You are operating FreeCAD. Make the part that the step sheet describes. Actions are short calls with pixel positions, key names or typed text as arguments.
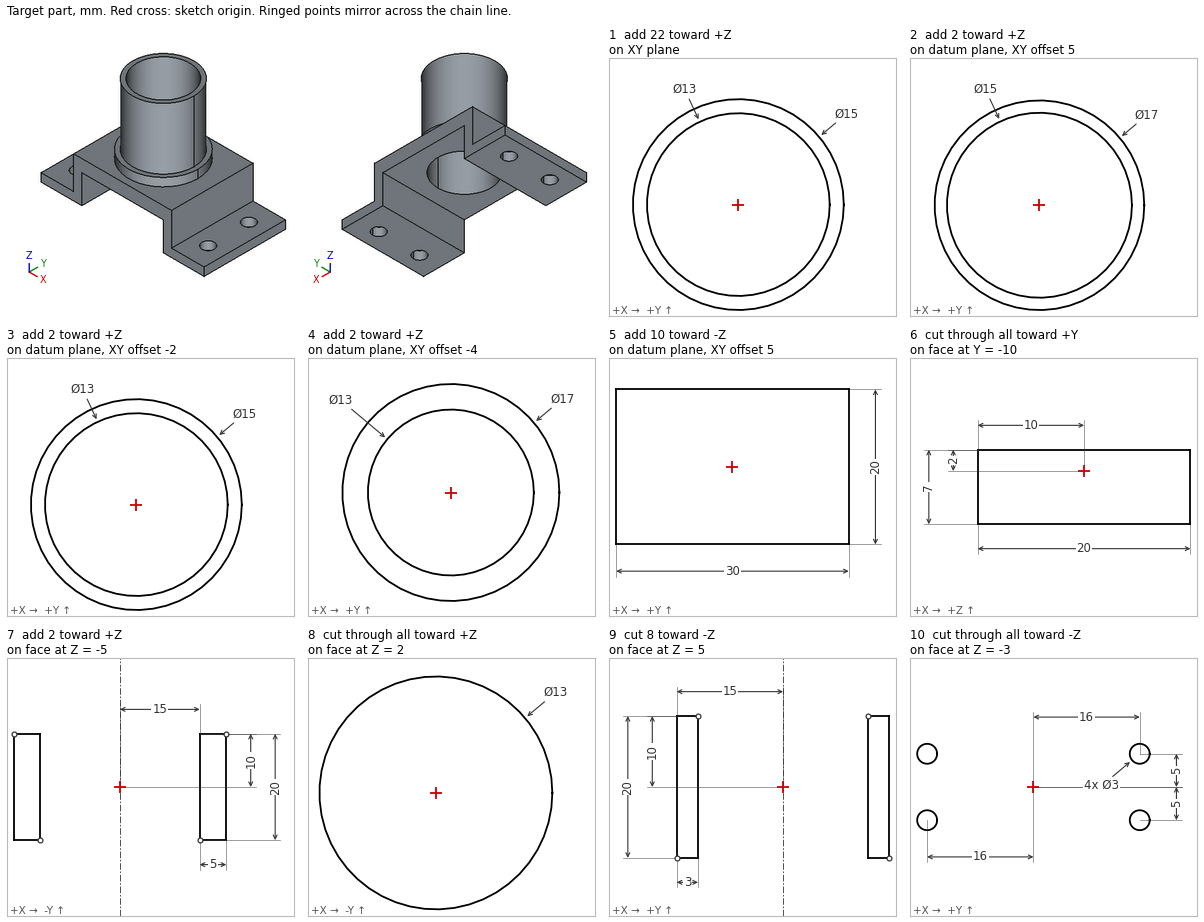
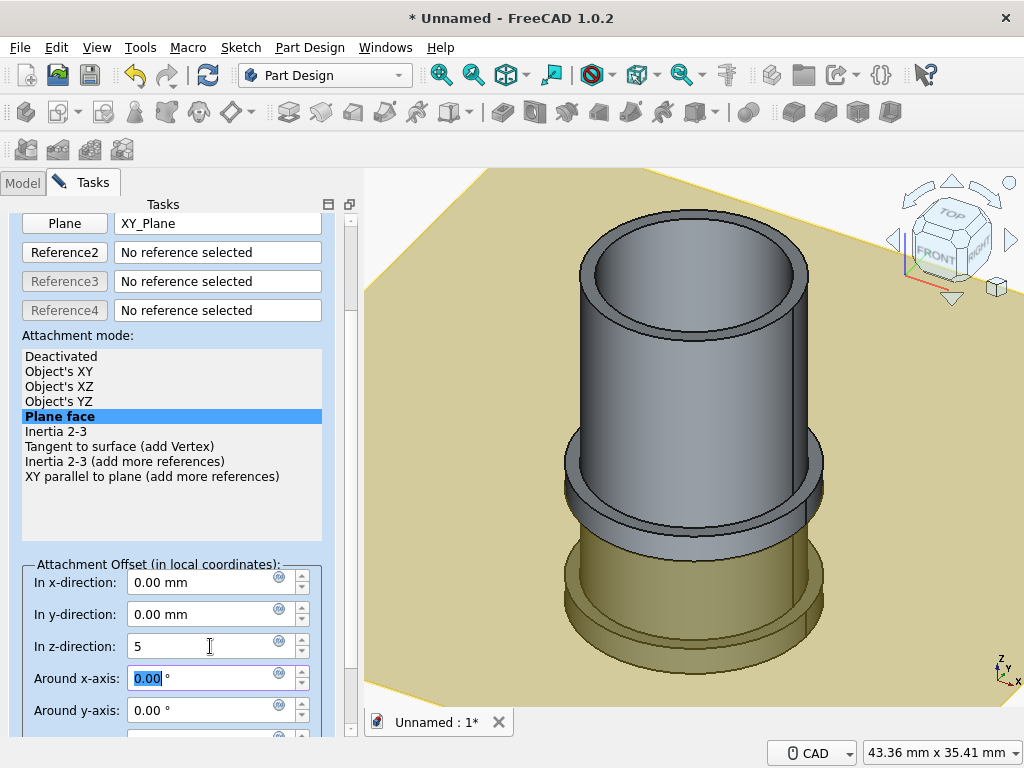
scroll(351, 475, up, 3)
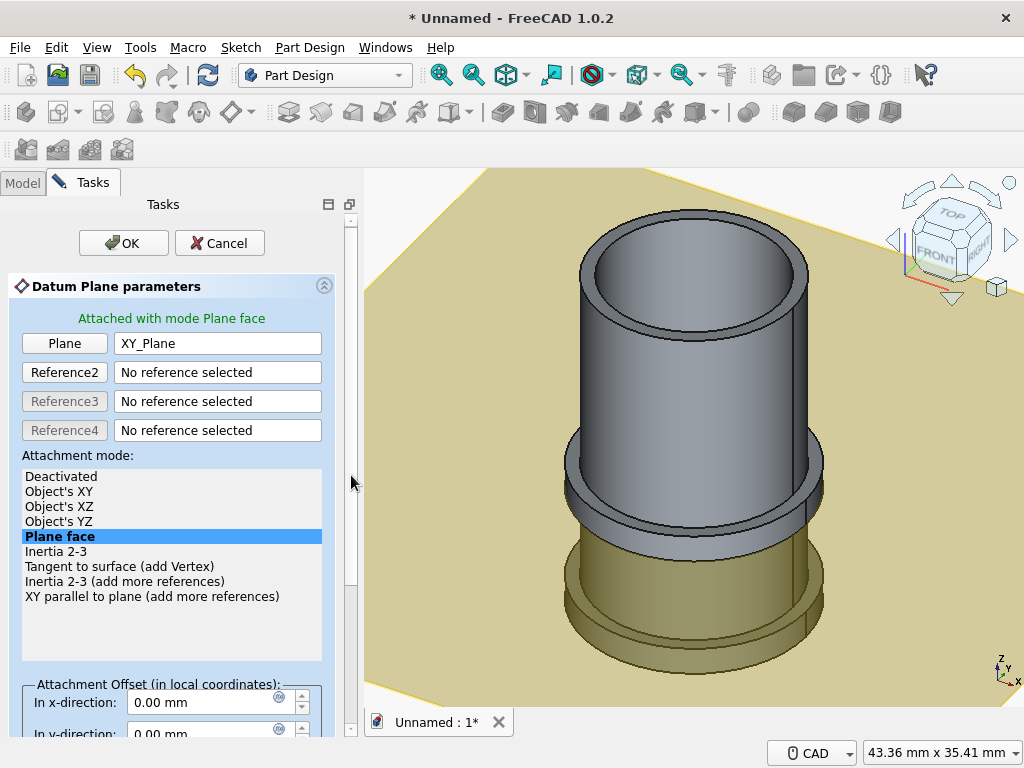
click(124, 243)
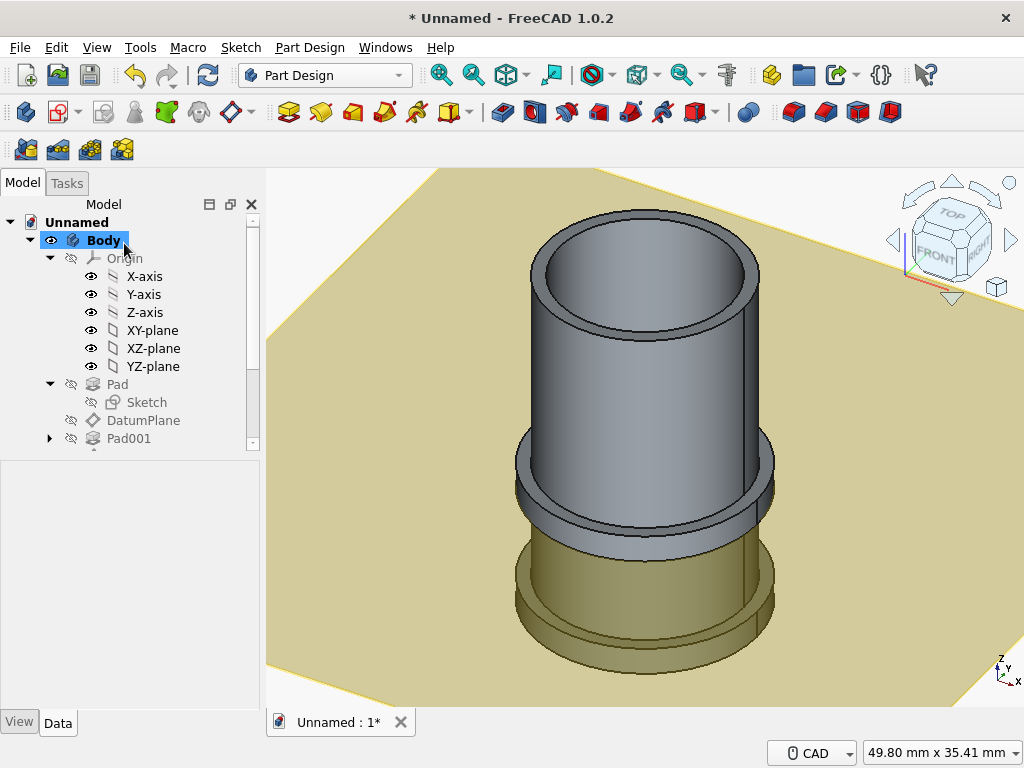
scroll(100, 326, down, 3)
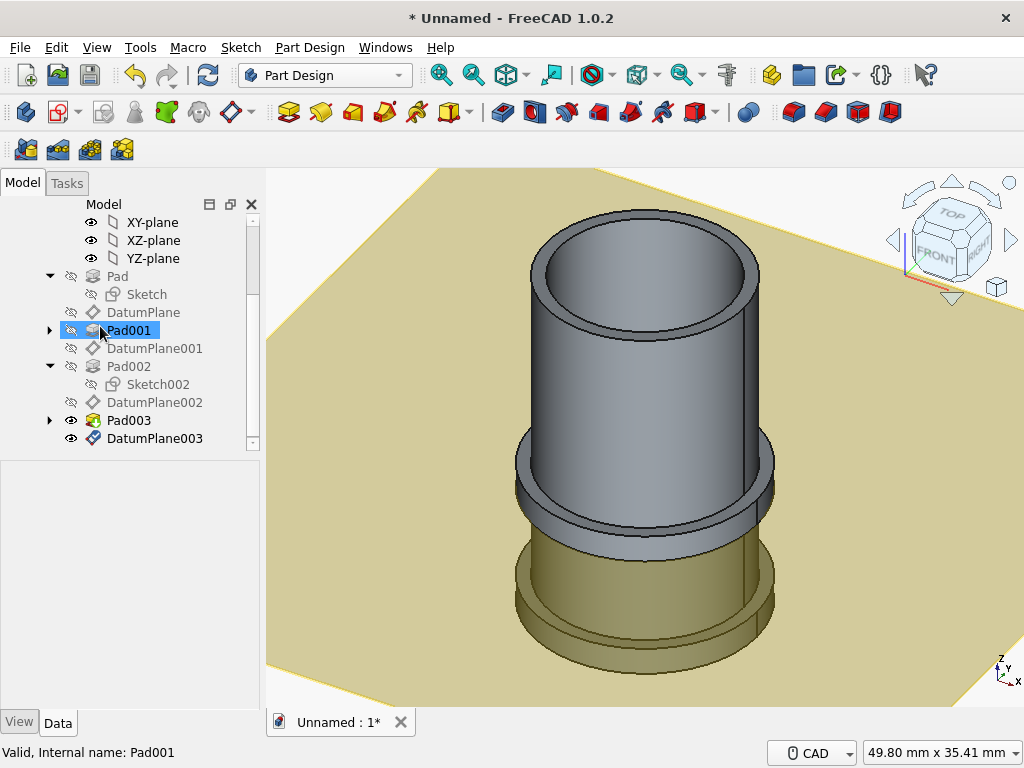
click(116, 438)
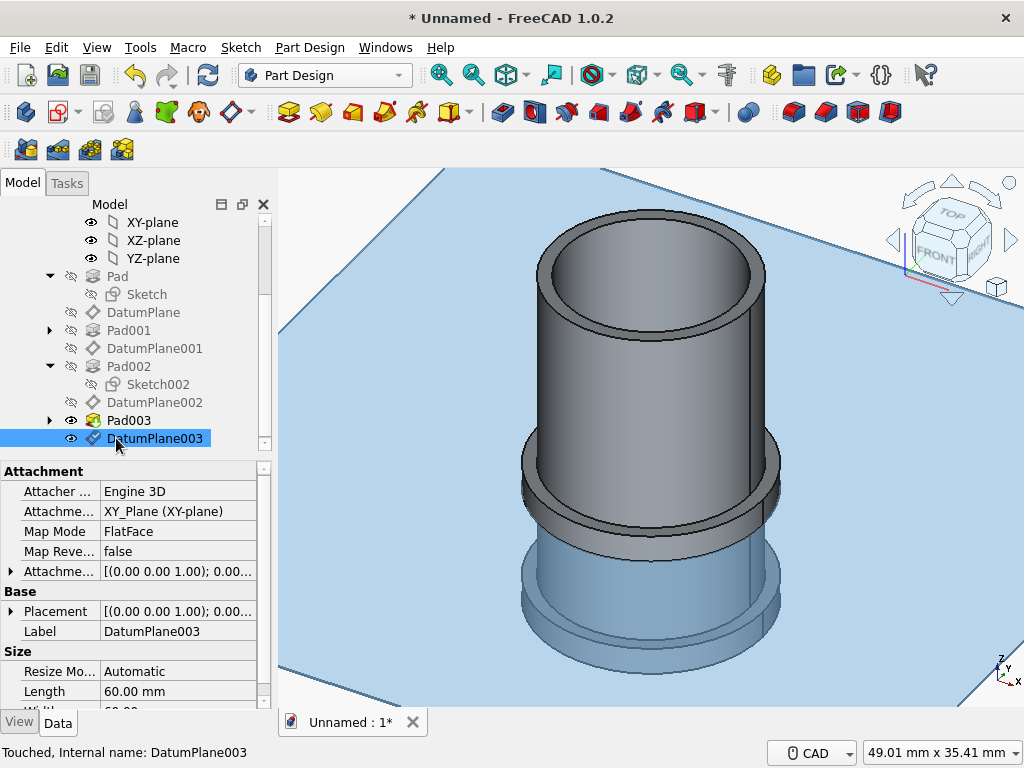
click(58, 112)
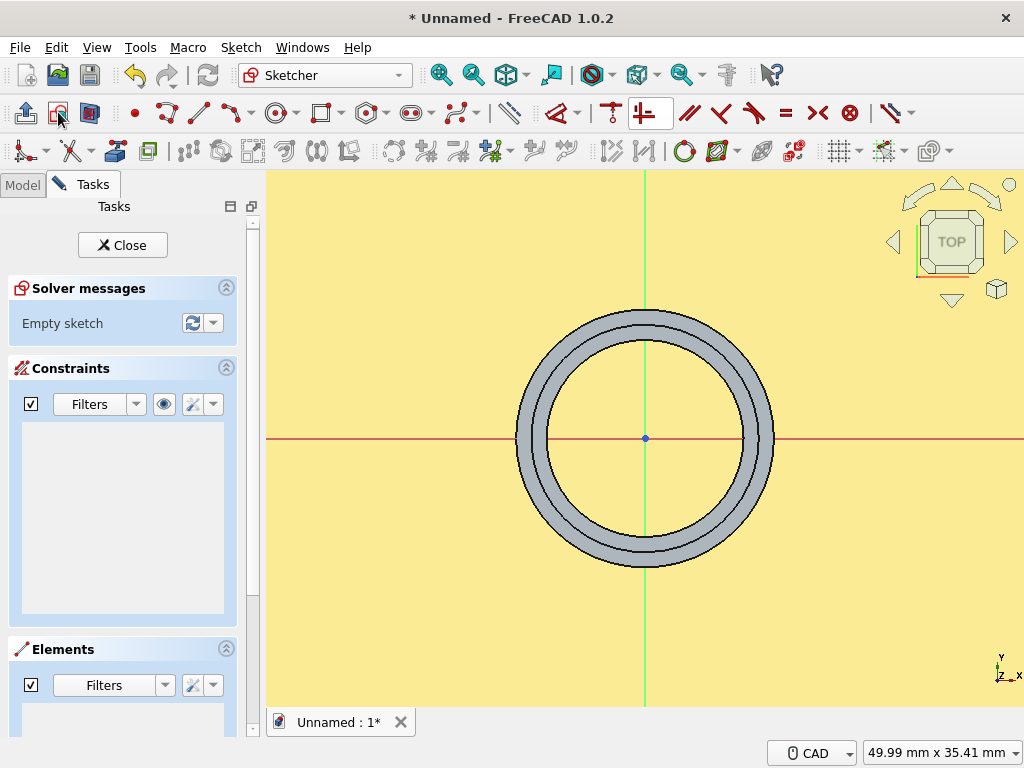
key(q)
key(s)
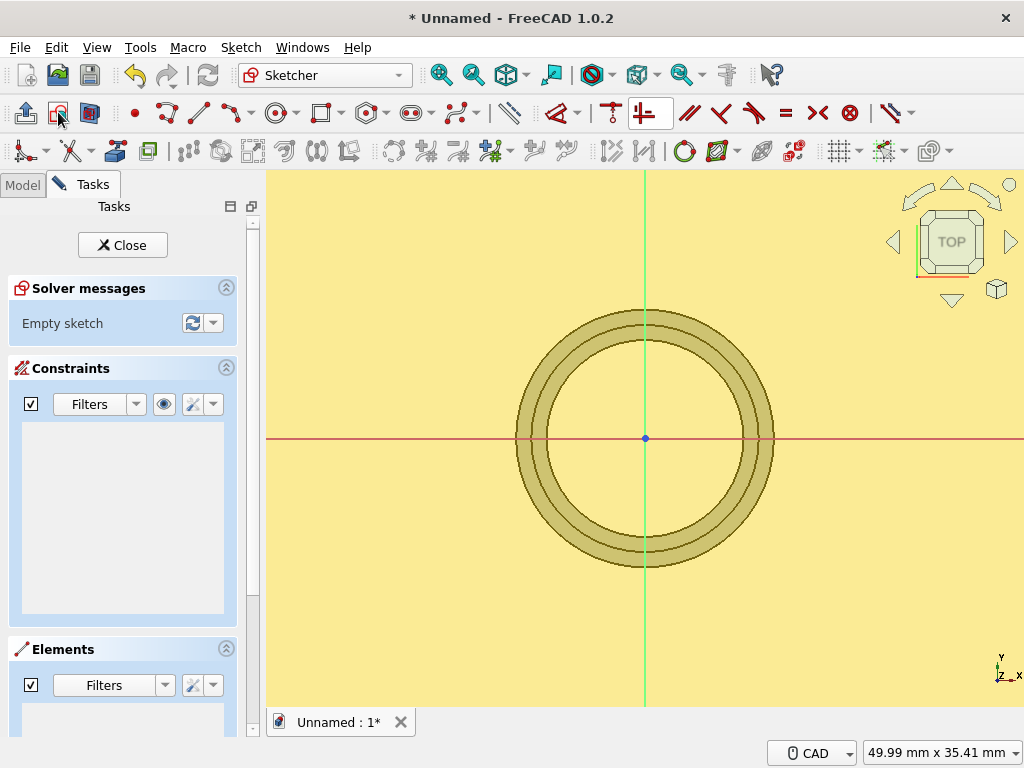
scroll(294, 439, down, 1)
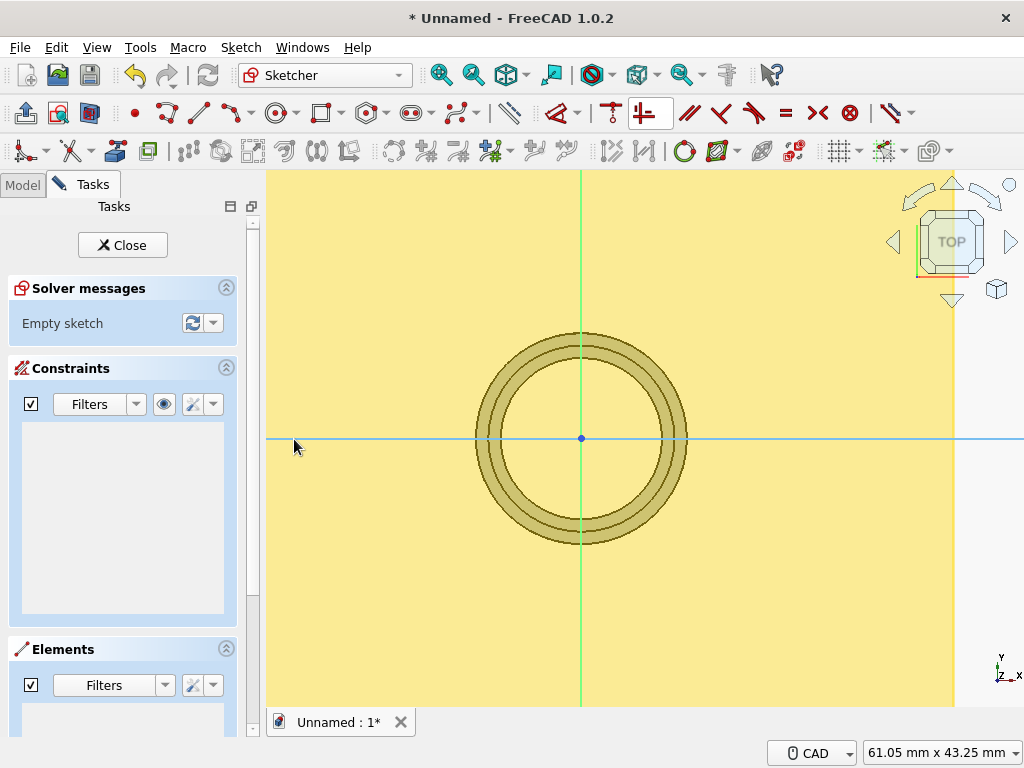
click(344, 114)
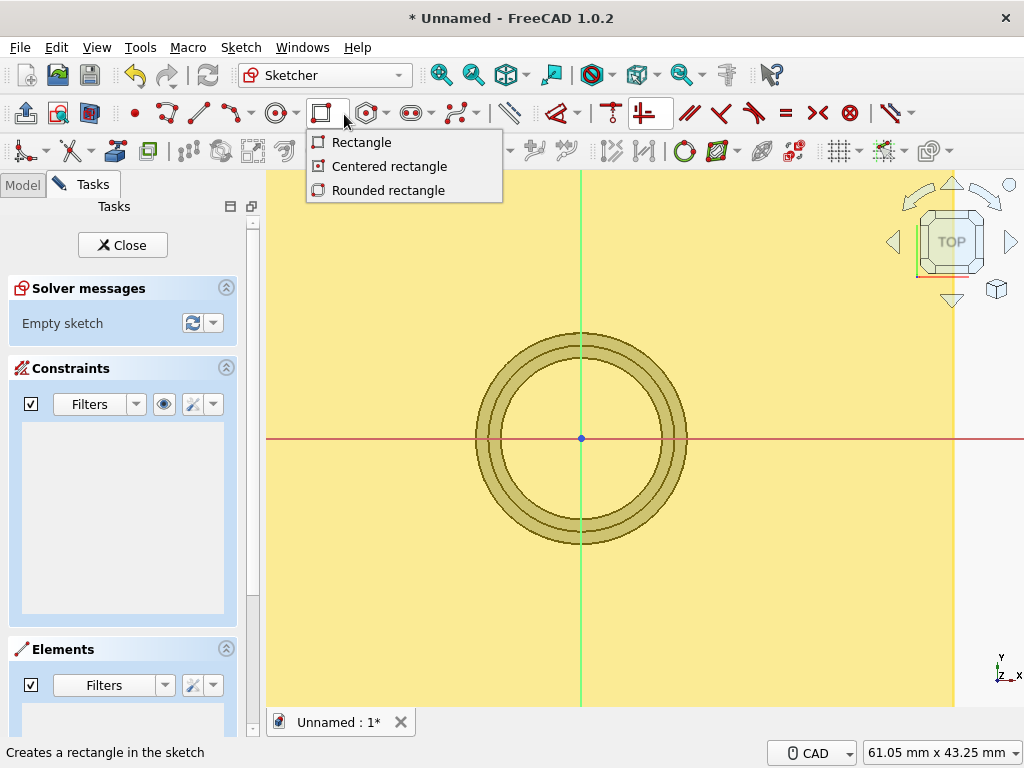
click(404, 166)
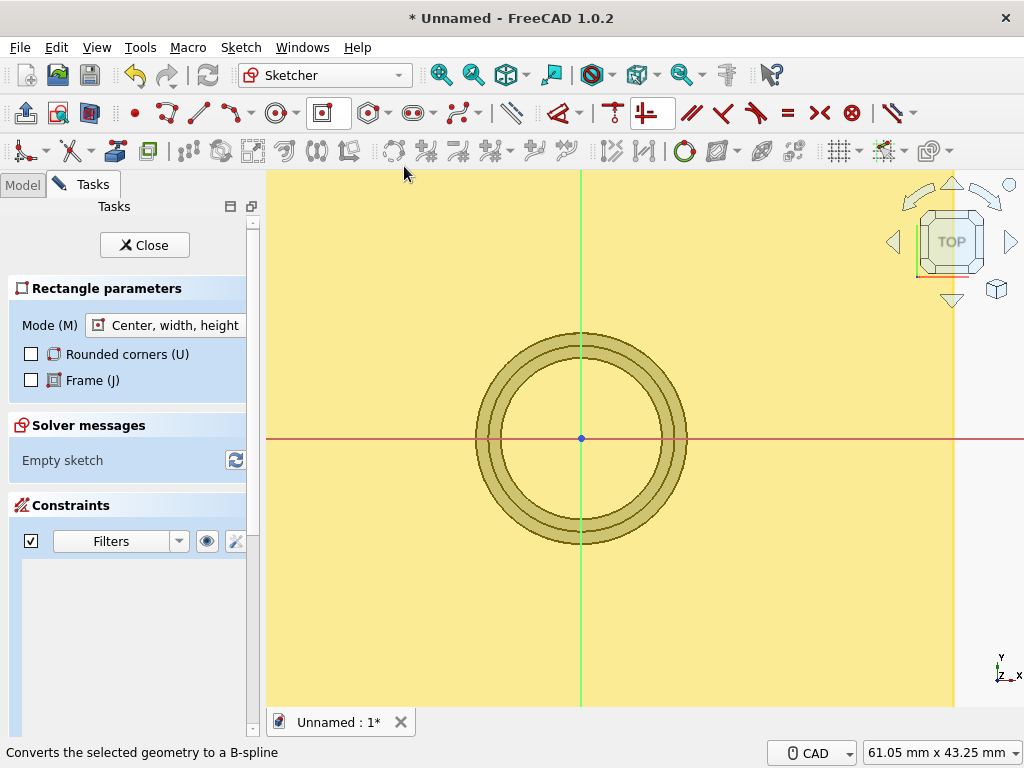
click(581, 439)
click(768, 315)
key(Escape)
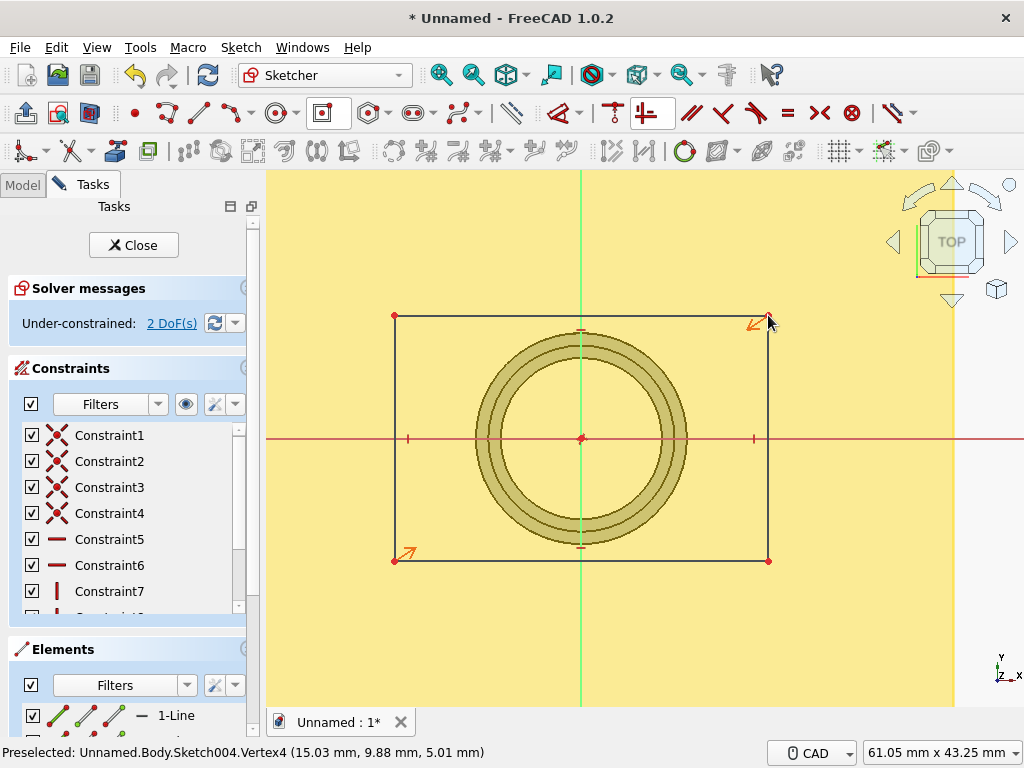
click(558, 114)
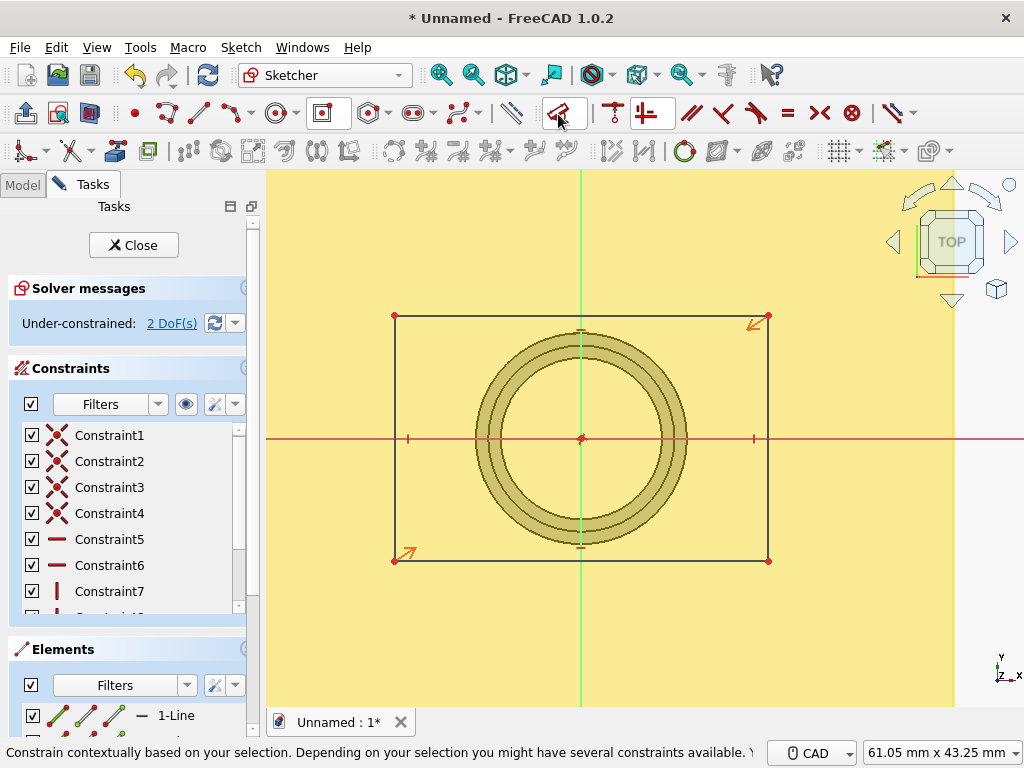
click(507, 561)
click(496, 595)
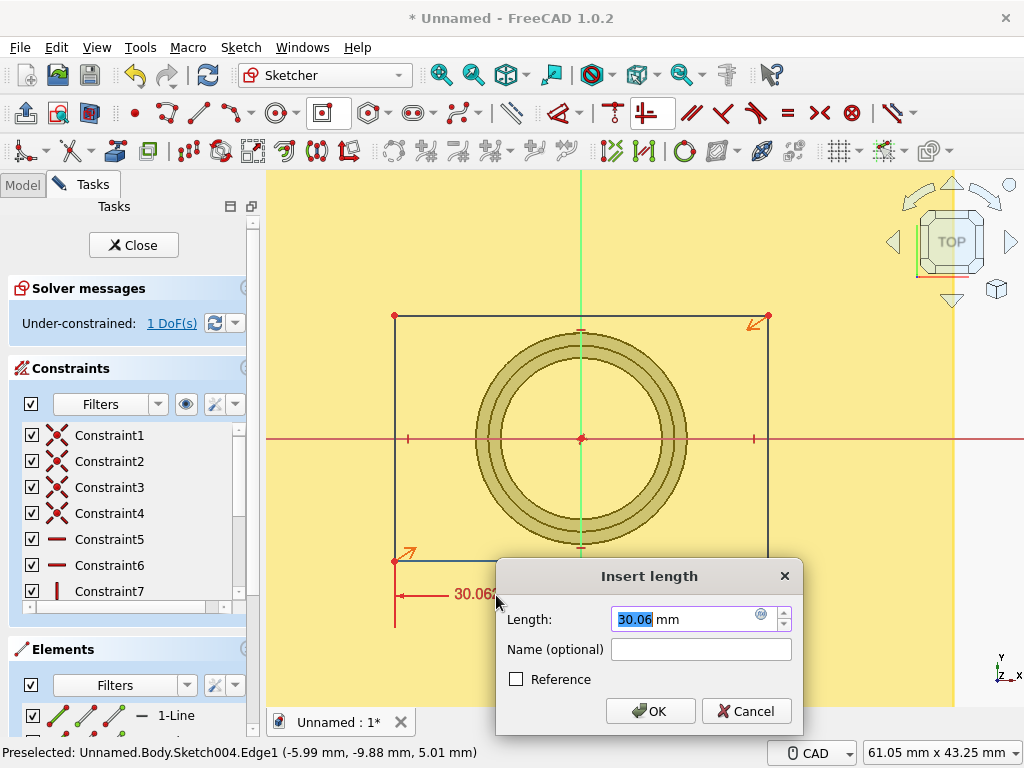
text(30)
key(Return)